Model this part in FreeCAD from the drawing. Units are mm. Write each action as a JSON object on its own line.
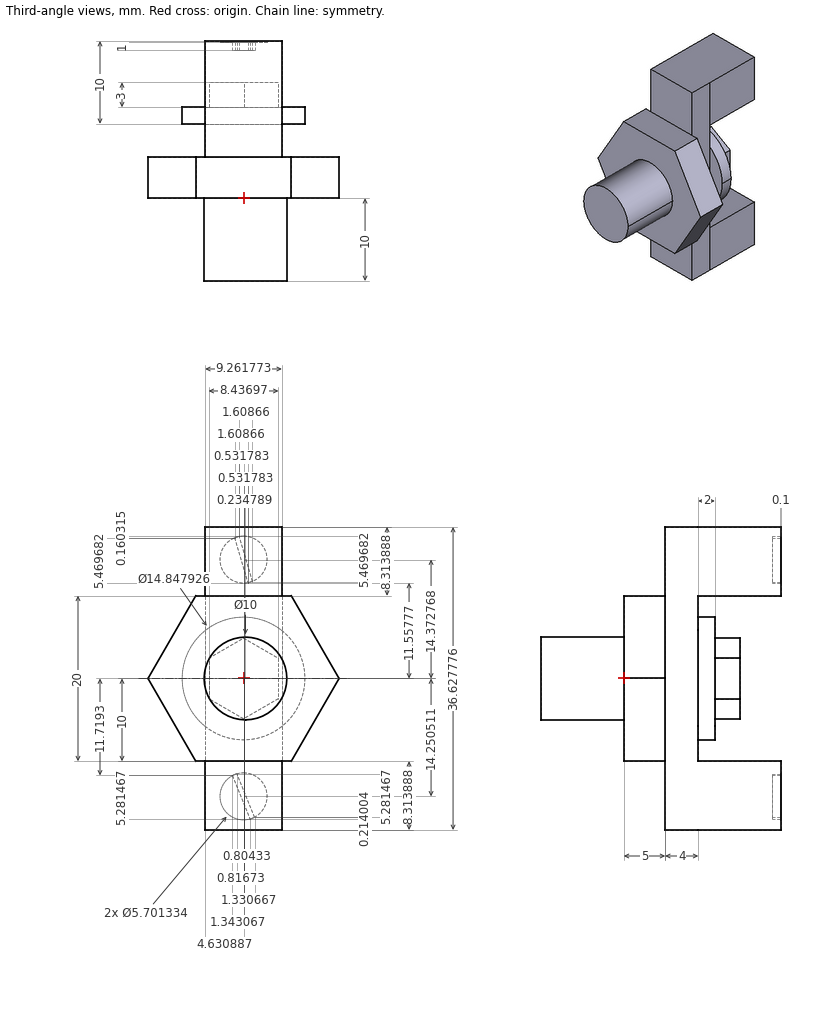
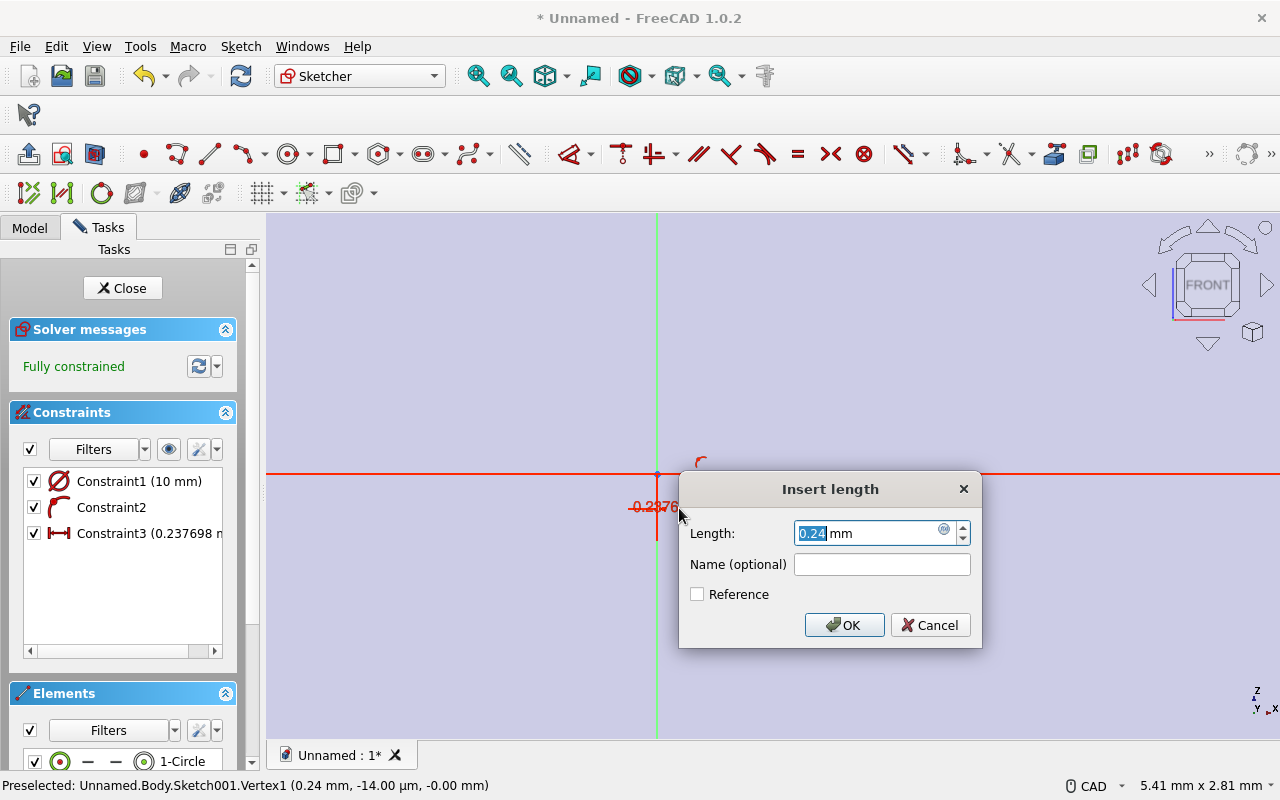
{"action": "type", "text": "0.234789"}
{"action": "key", "text": "Return"}
{"action": "key", "text": "Escape"}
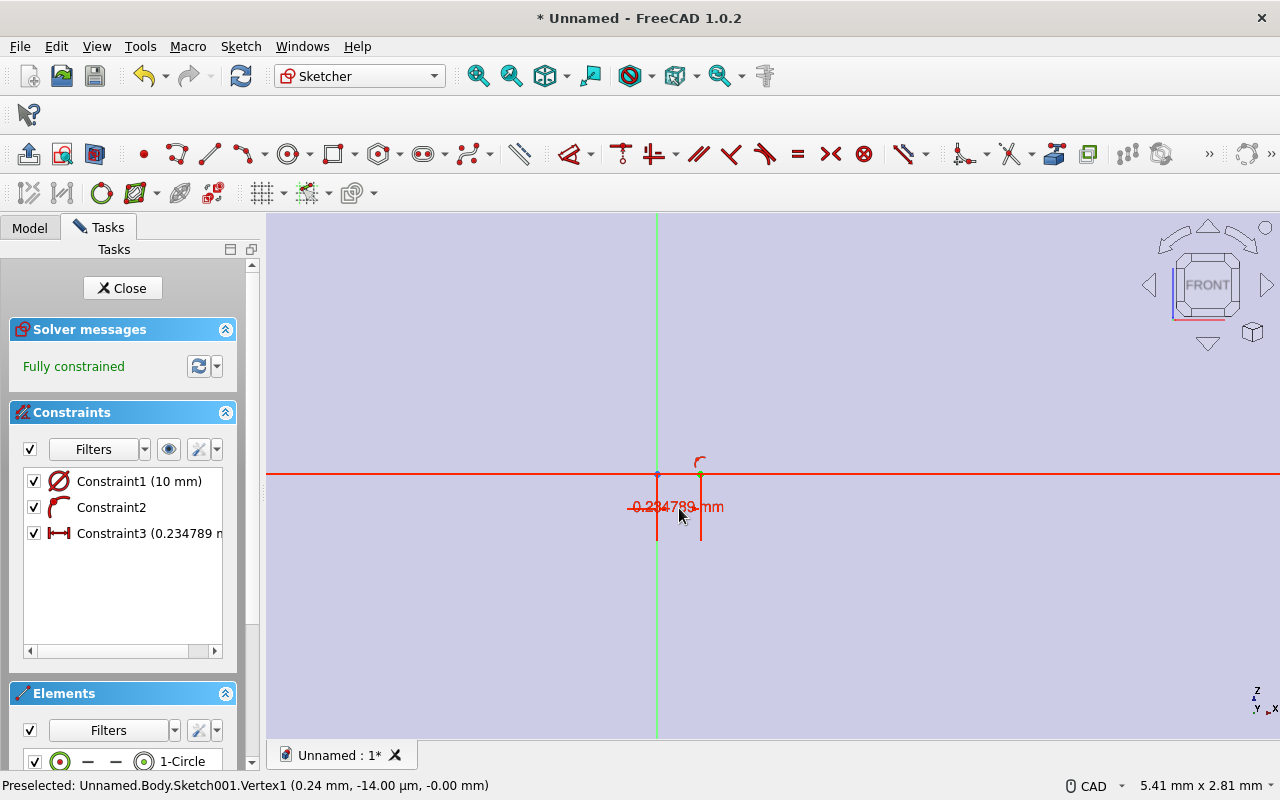
{"action": "left_click", "coordinate": [123, 288]}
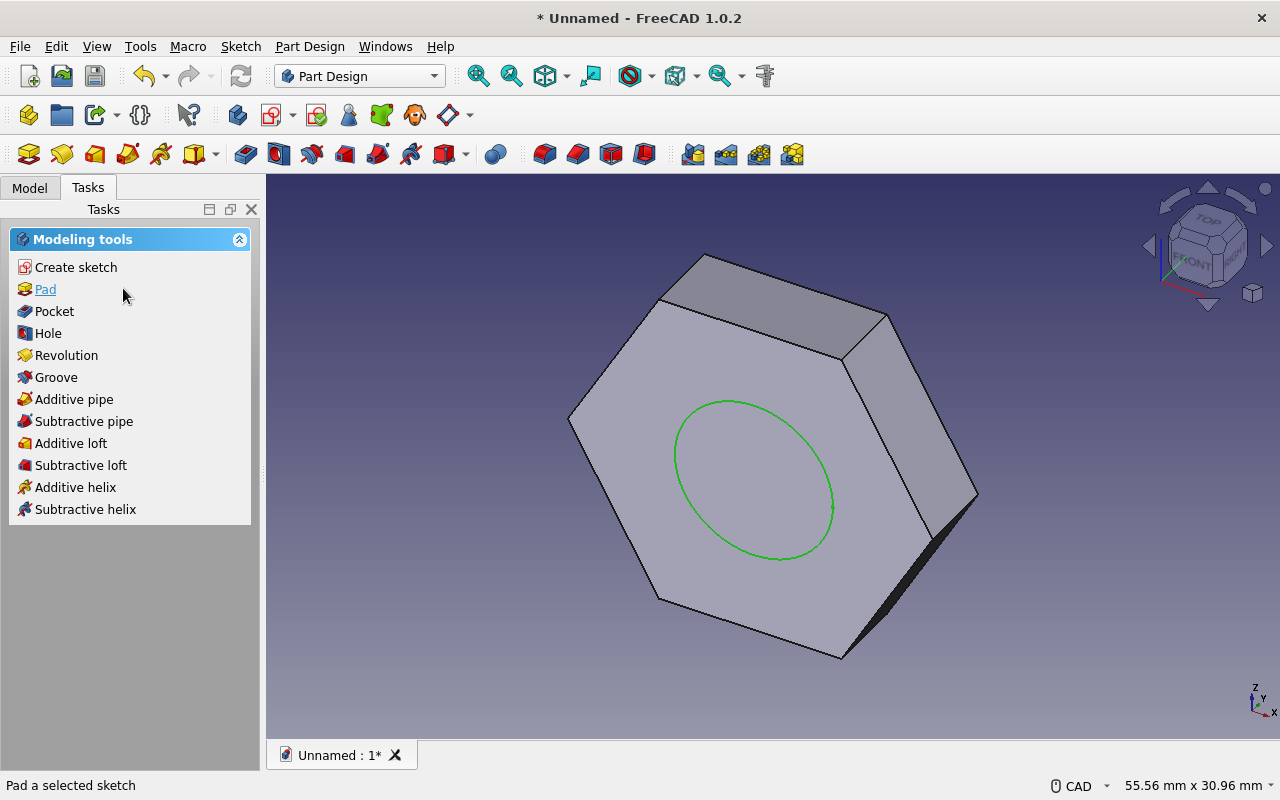
{"action": "left_click", "coordinate": [29, 154]}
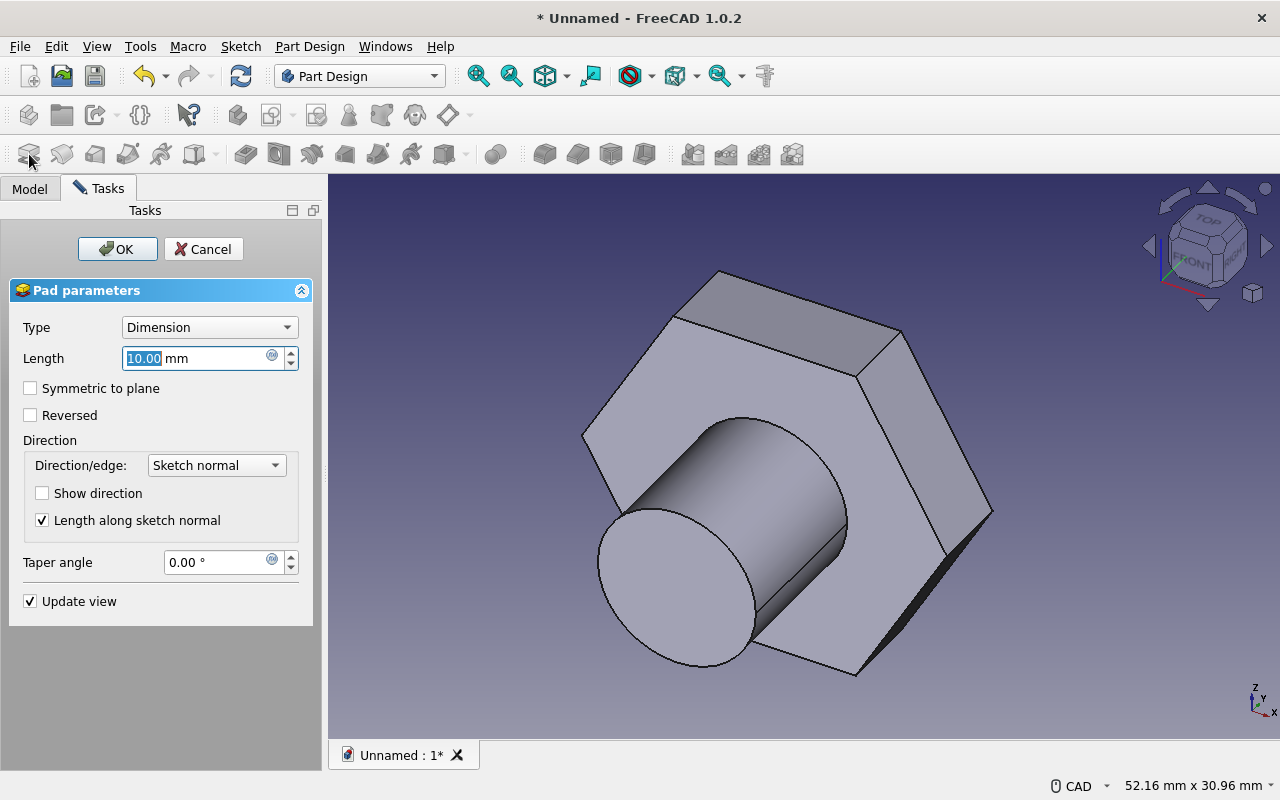
{"action": "type", "text": "10"}
{"action": "key", "text": "Tab"}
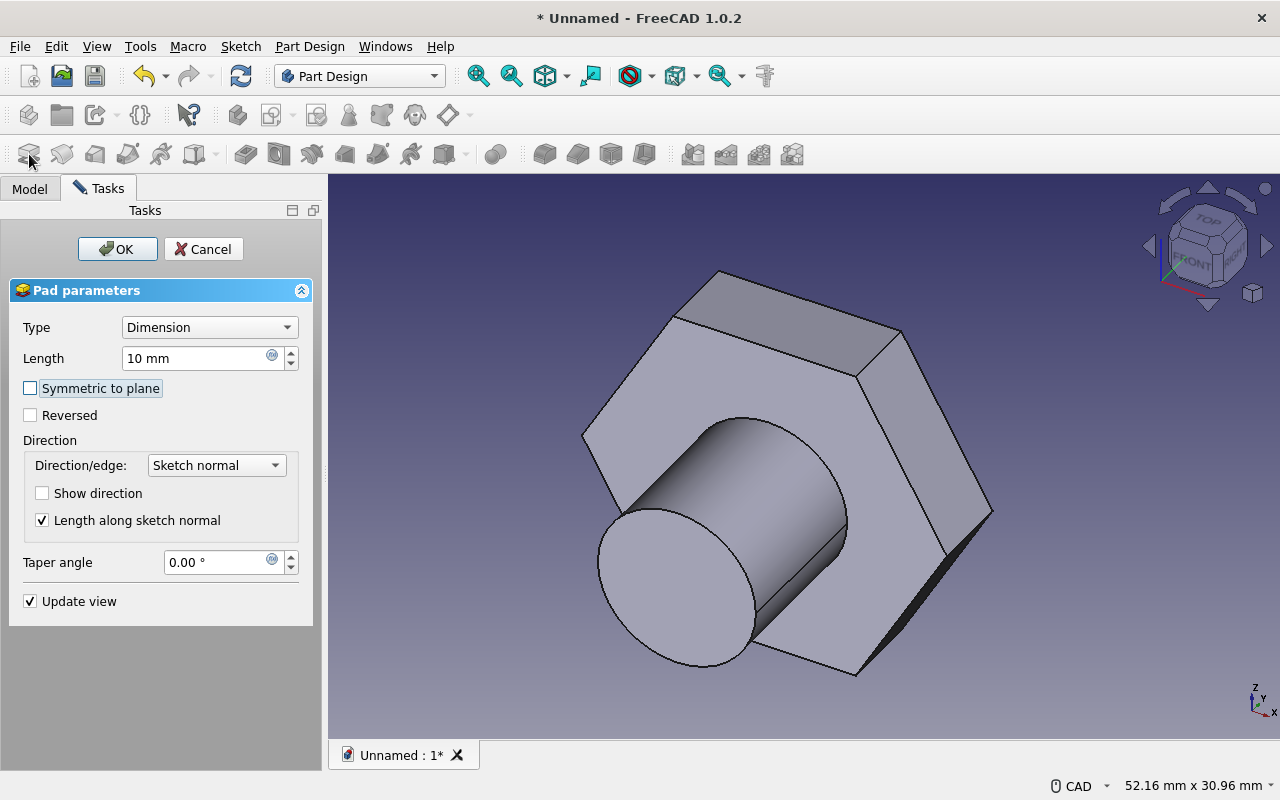
{"action": "left_click", "coordinate": [118, 249]}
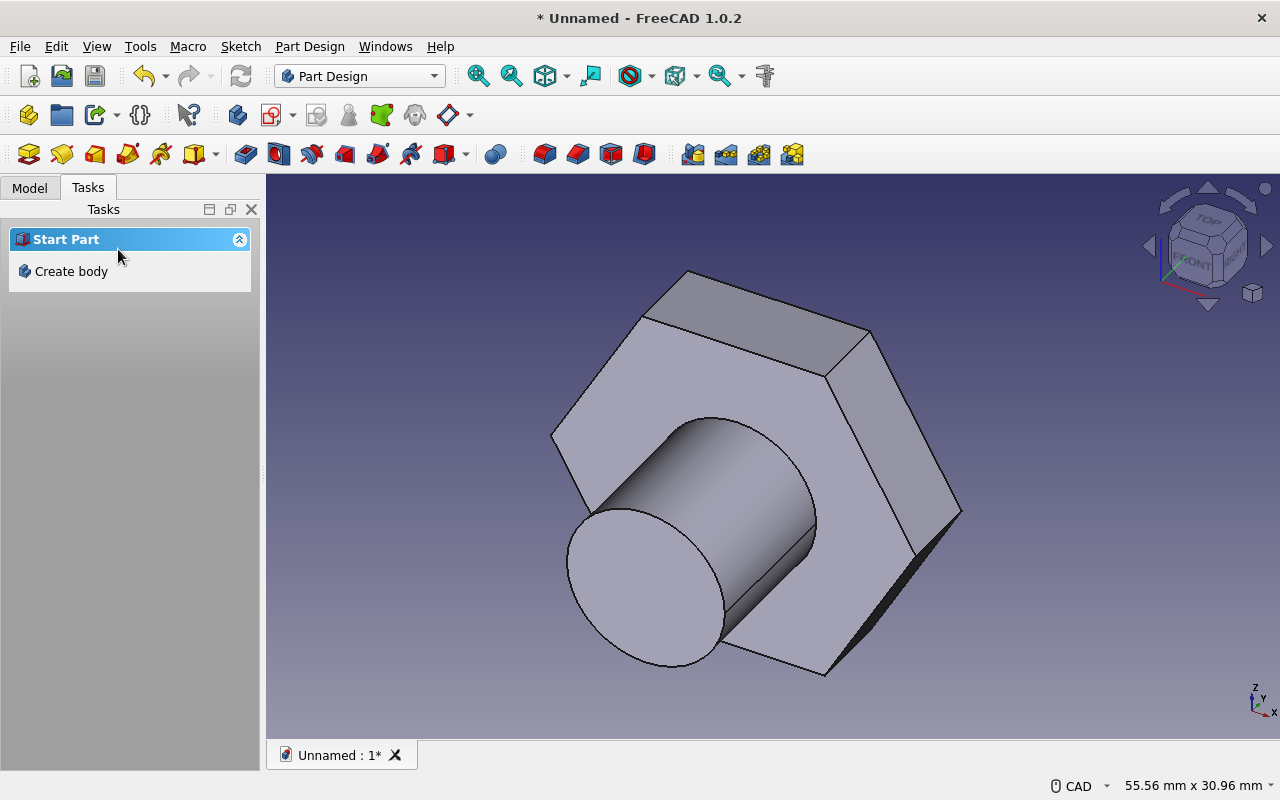
{"action": "left_click", "coordinate": [479, 76]}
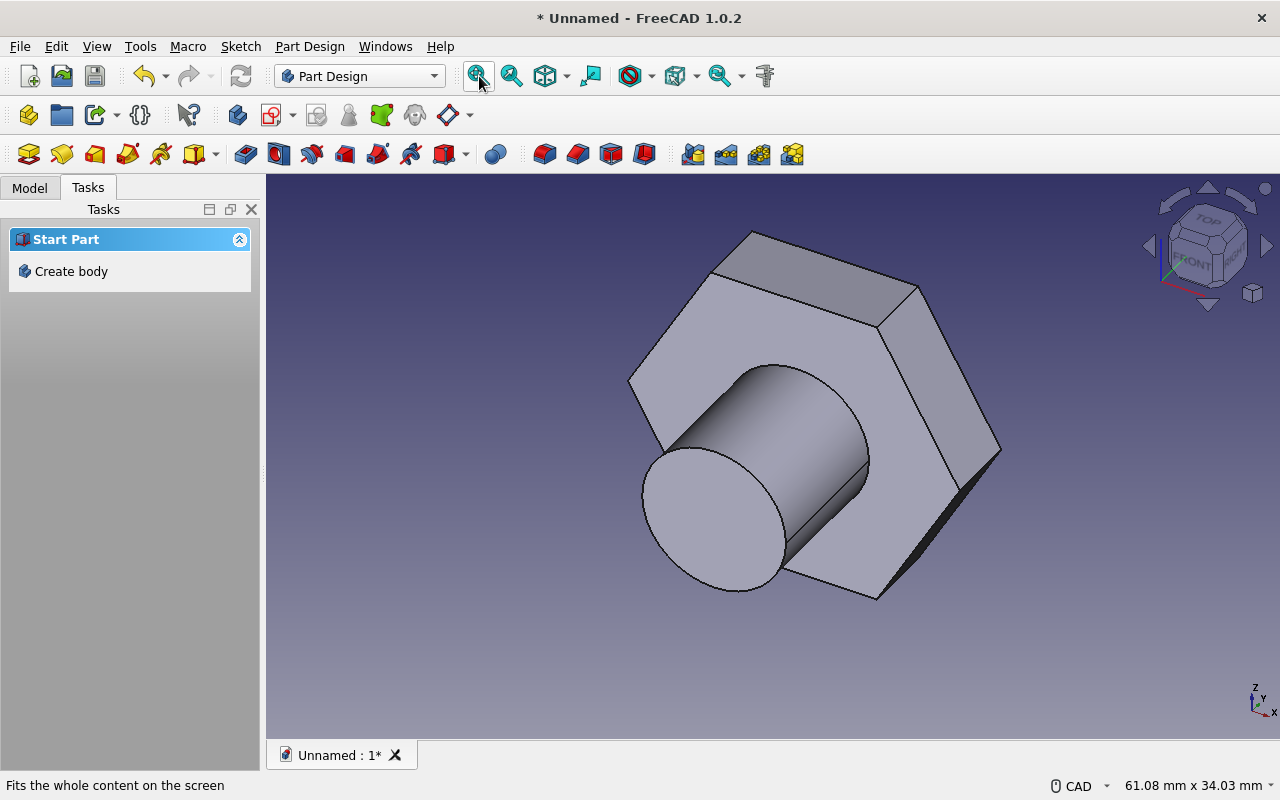
{"action": "key", "text": "4"}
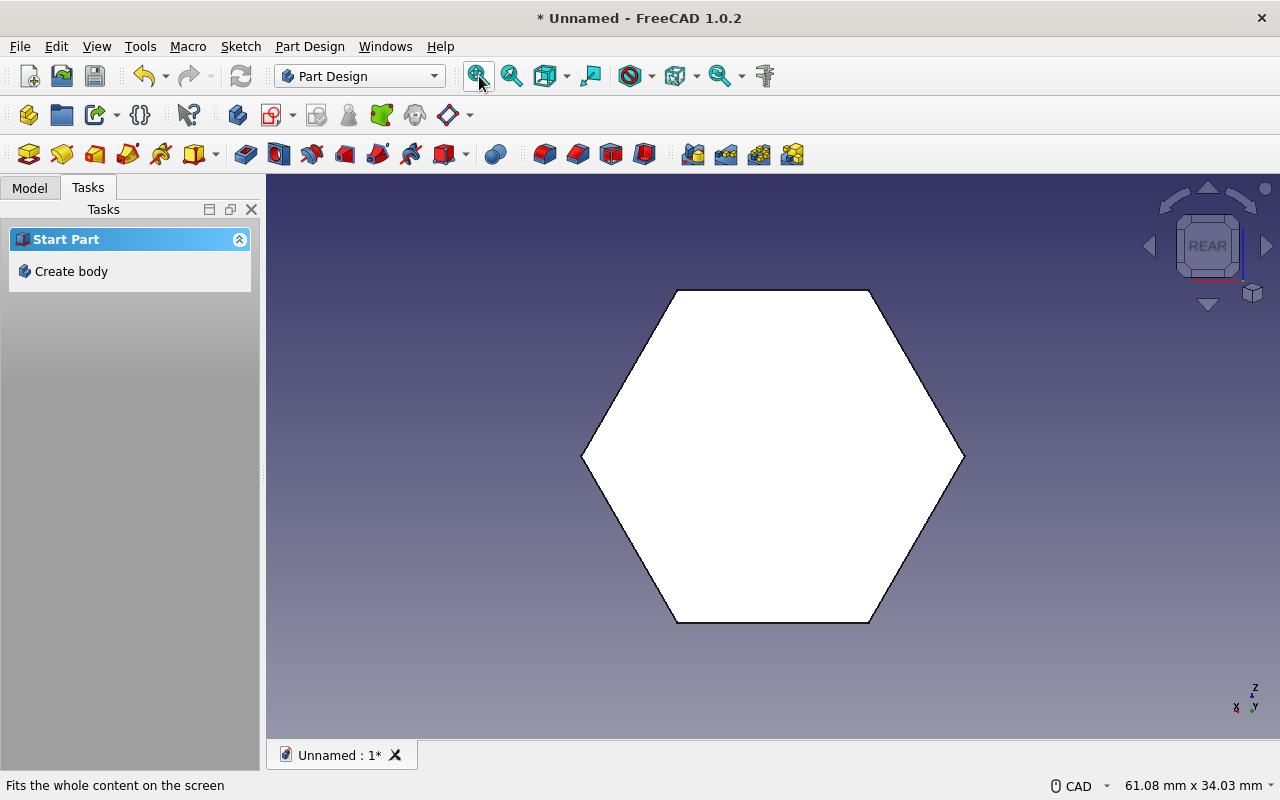
{"action": "left_click", "coordinate": [773, 455]}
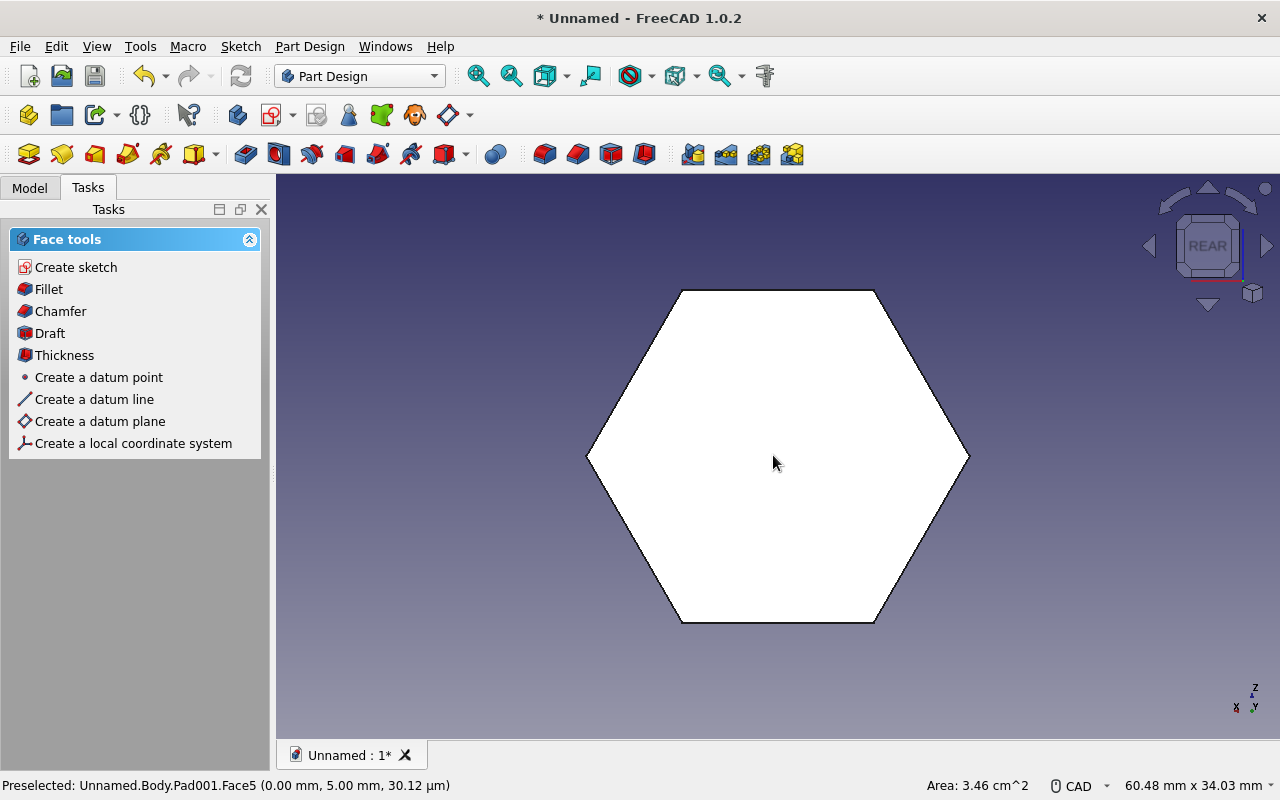
{"action": "left_click", "coordinate": [270, 116]}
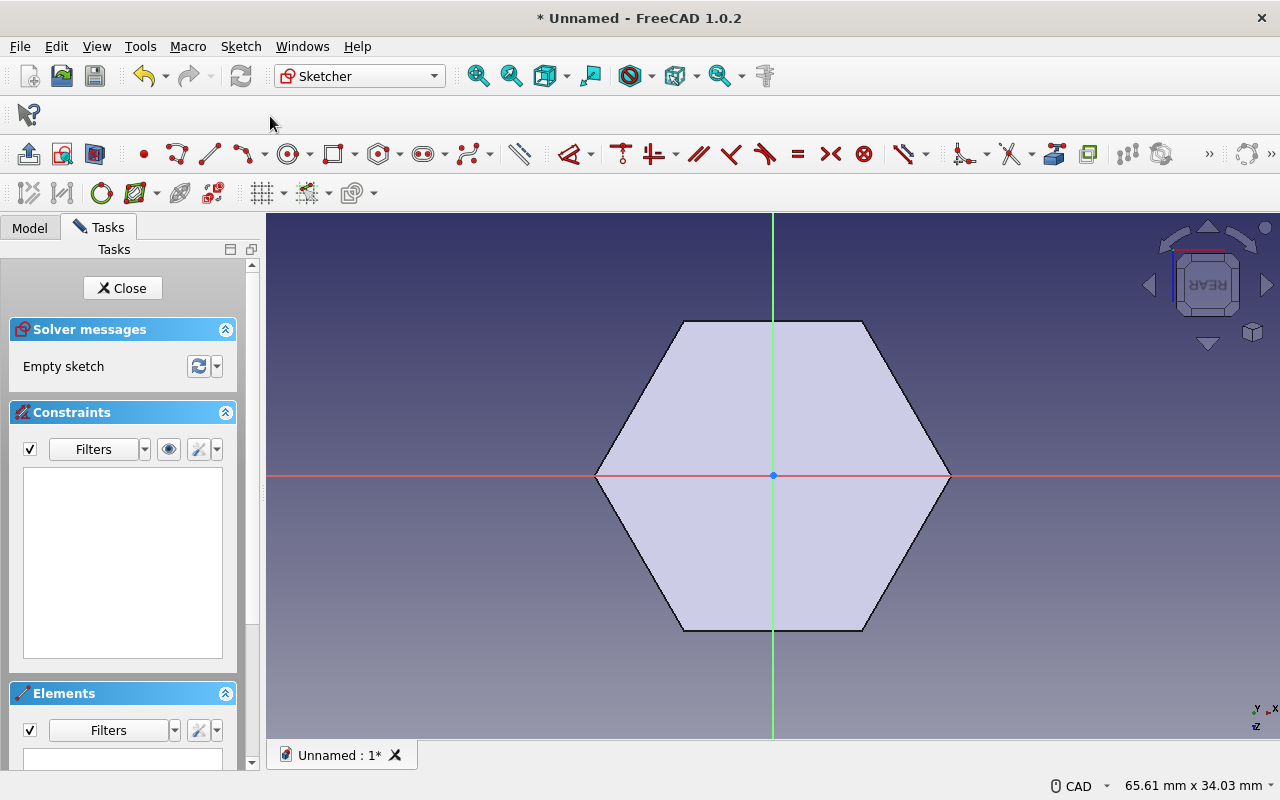
{"action": "scroll", "coordinate": [621, 476], "scroll_direction": "down", "scroll_amount": 3}